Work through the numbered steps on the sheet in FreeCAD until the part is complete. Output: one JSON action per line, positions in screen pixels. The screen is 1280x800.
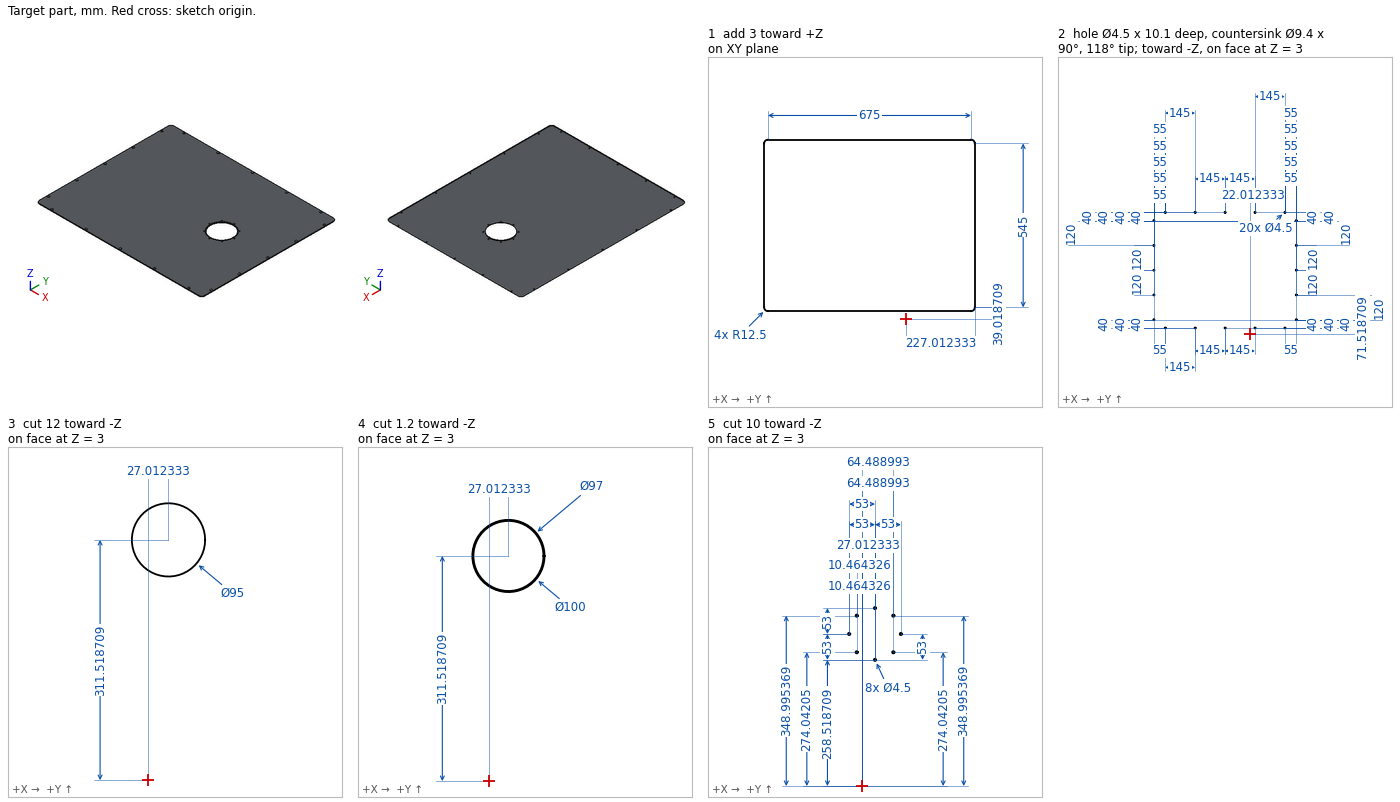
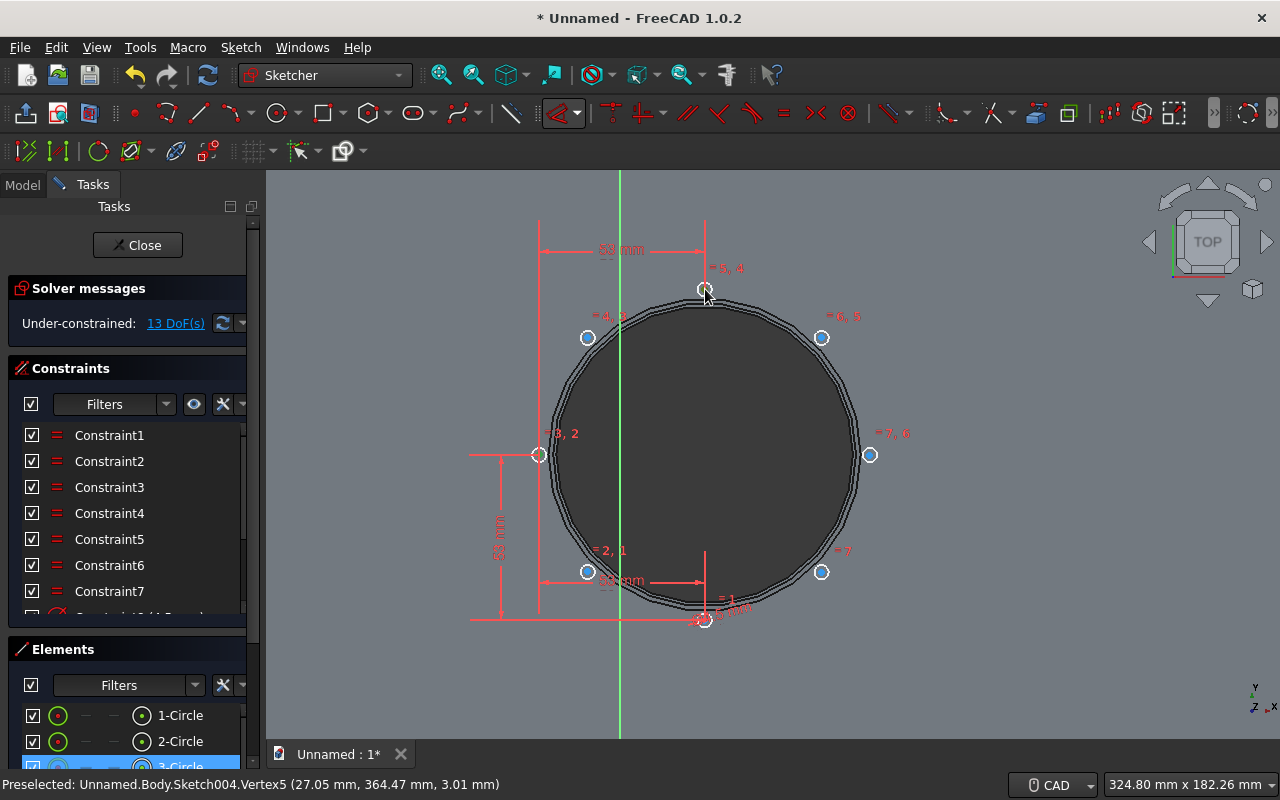
{"action": "left_click", "coordinate": [580, 114]}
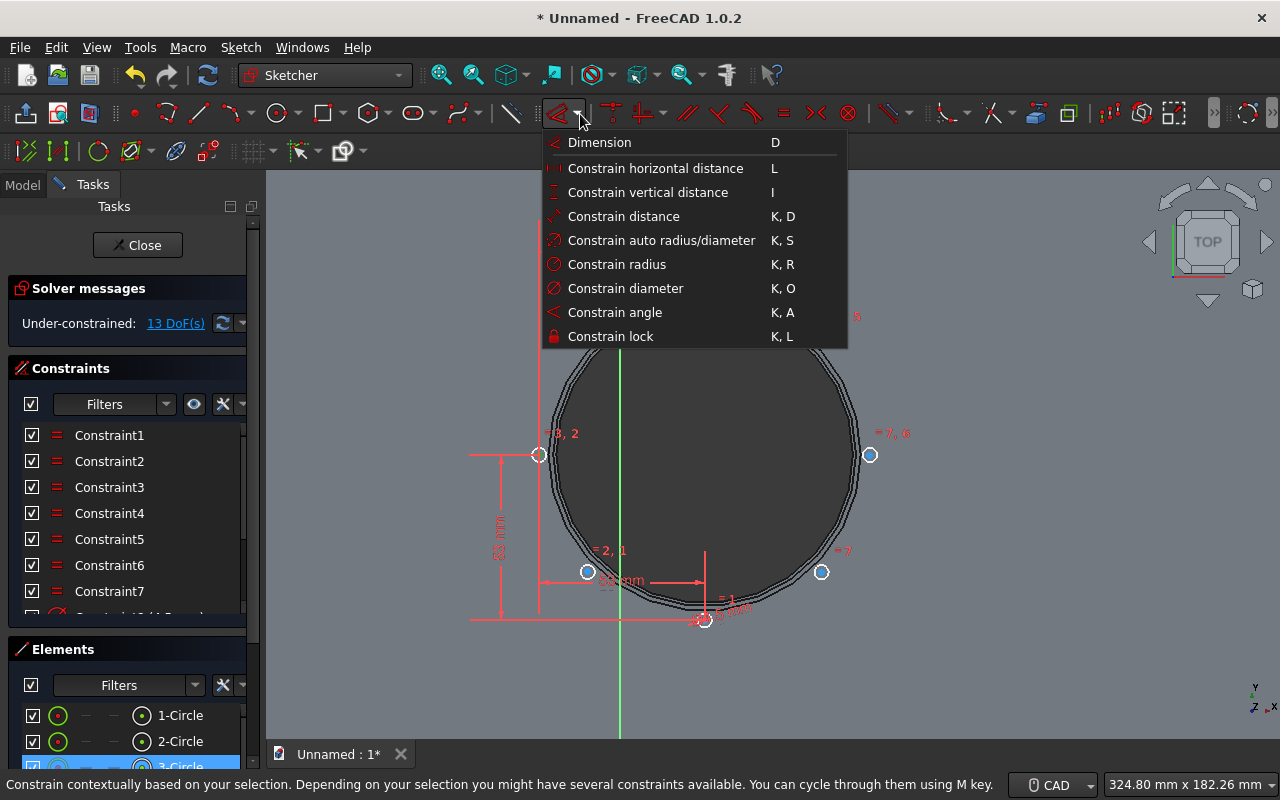
{"action": "left_click", "coordinate": [695, 192]}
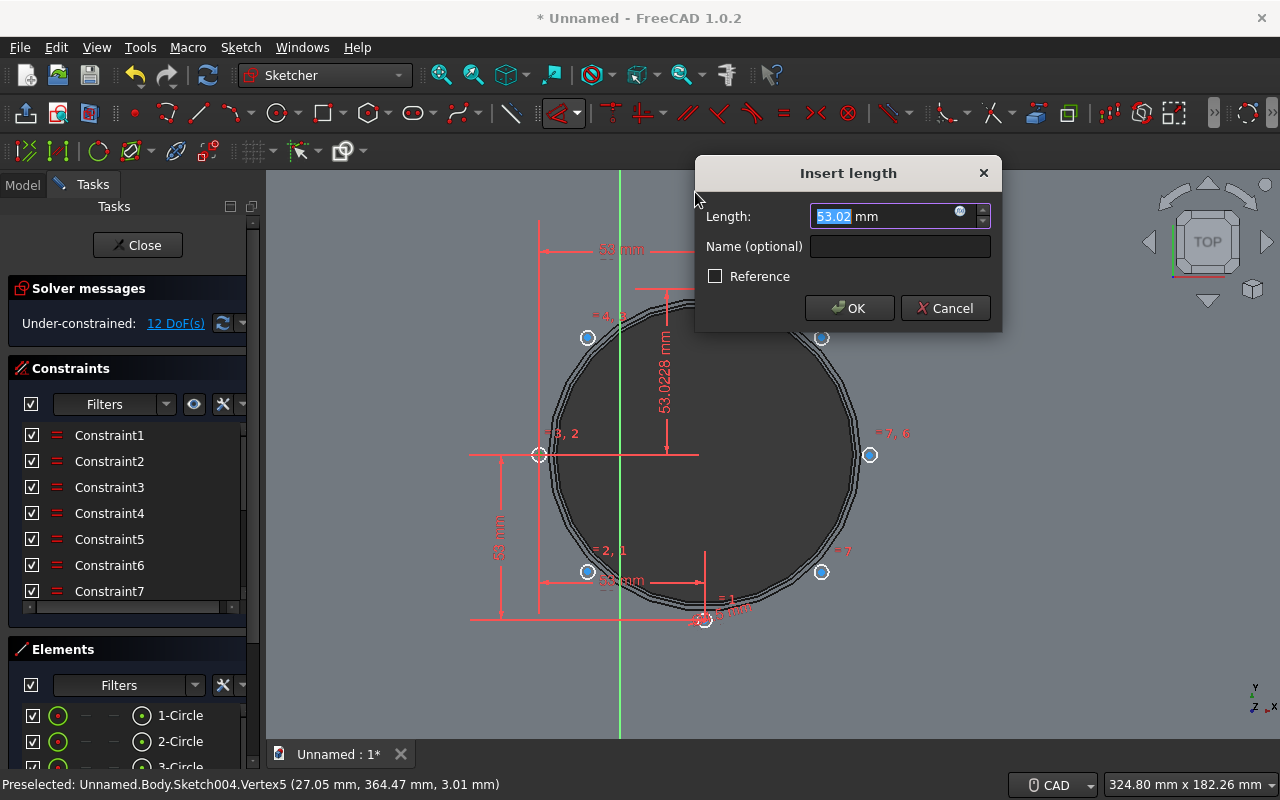
{"action": "type", "text": "53"}
{"action": "key", "text": "Return"}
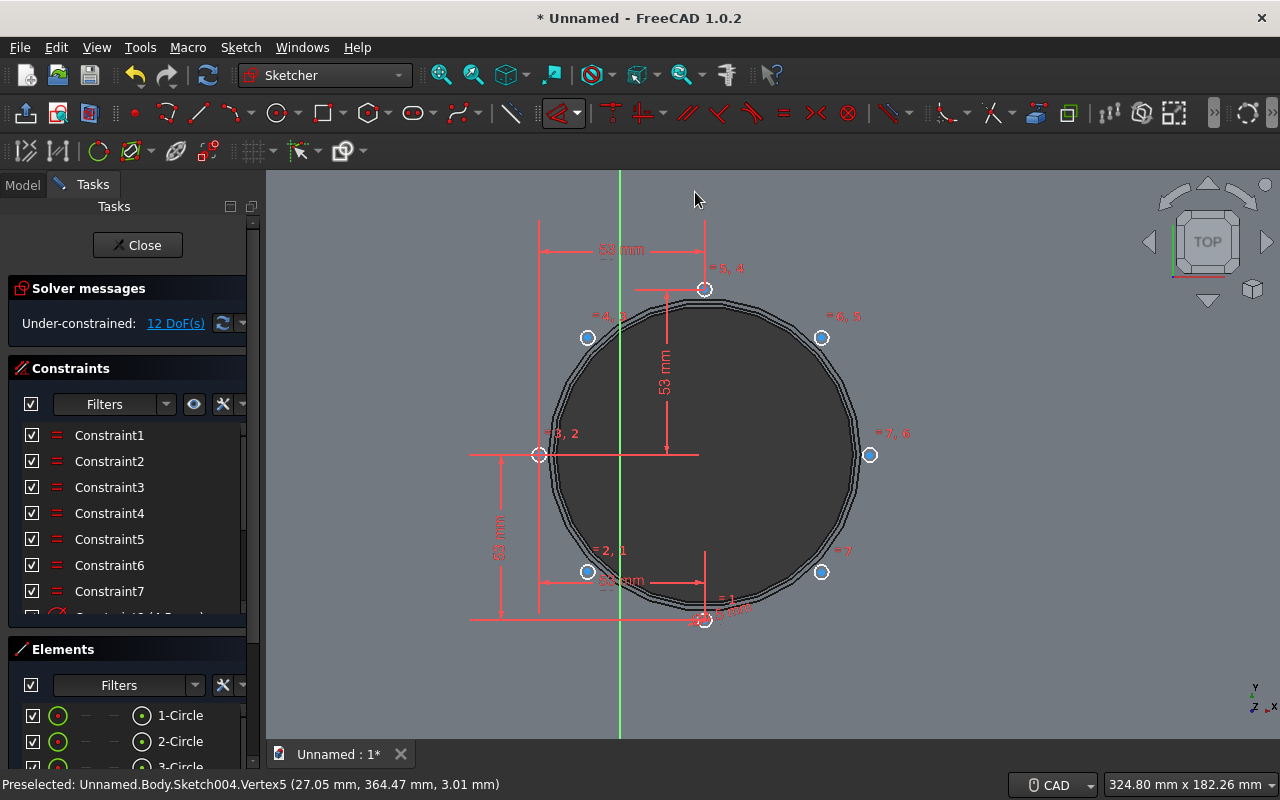
{"action": "left_click", "coordinate": [705, 620]}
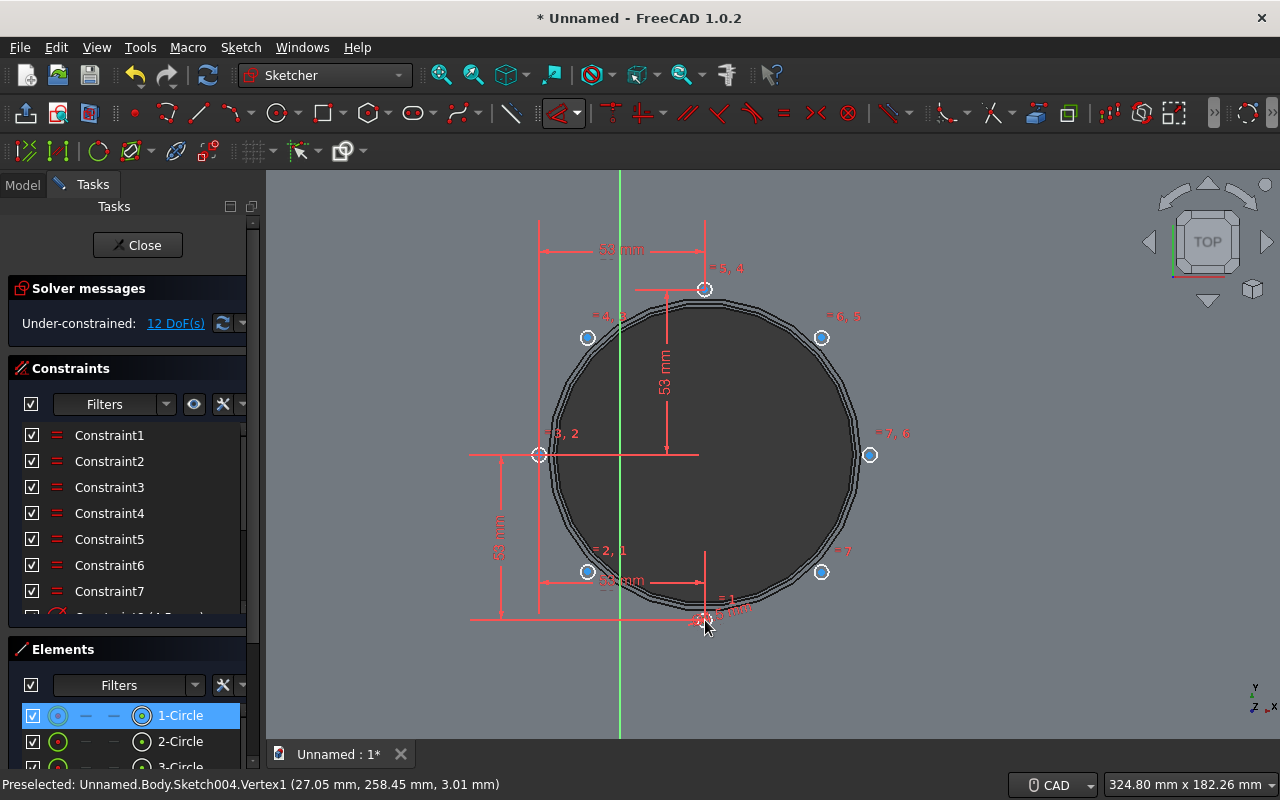
{"action": "left_click", "coordinate": [870, 455]}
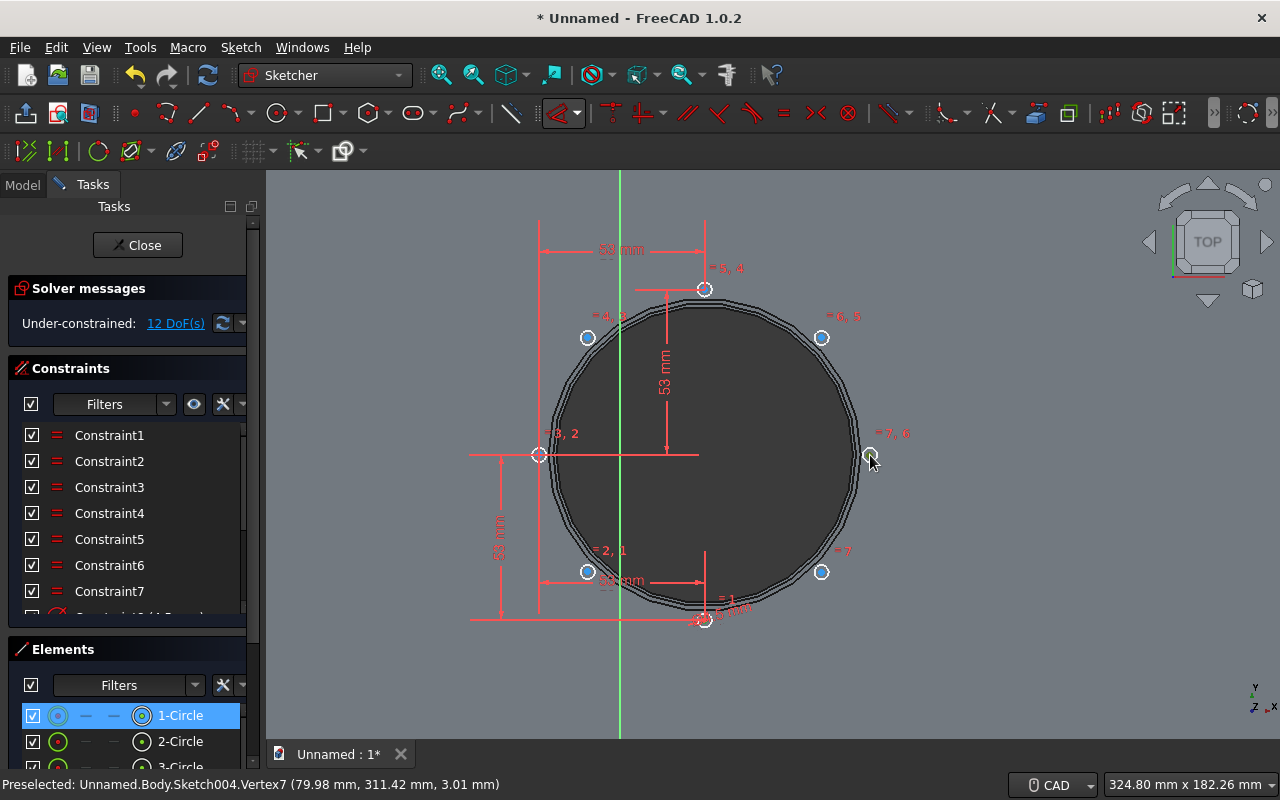
{"action": "left_click", "coordinate": [580, 114]}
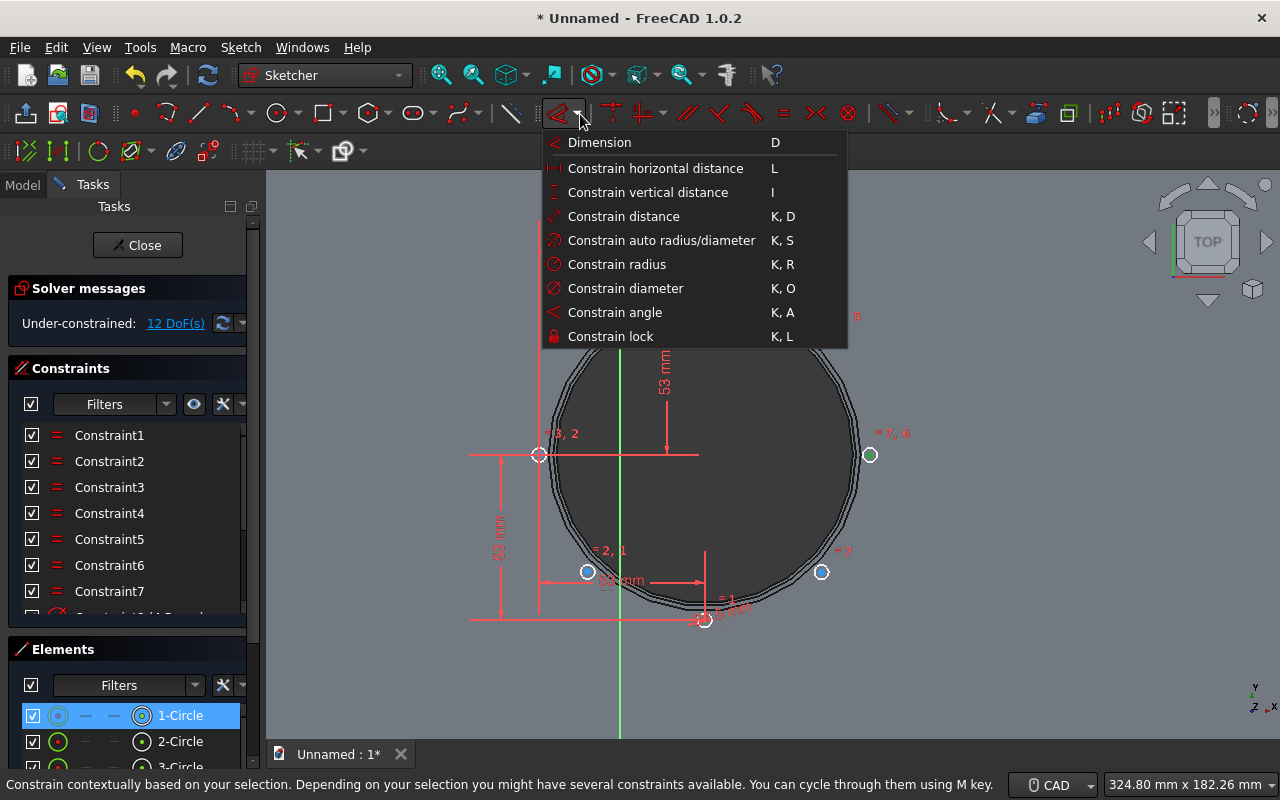
{"action": "left_click", "coordinate": [695, 168]}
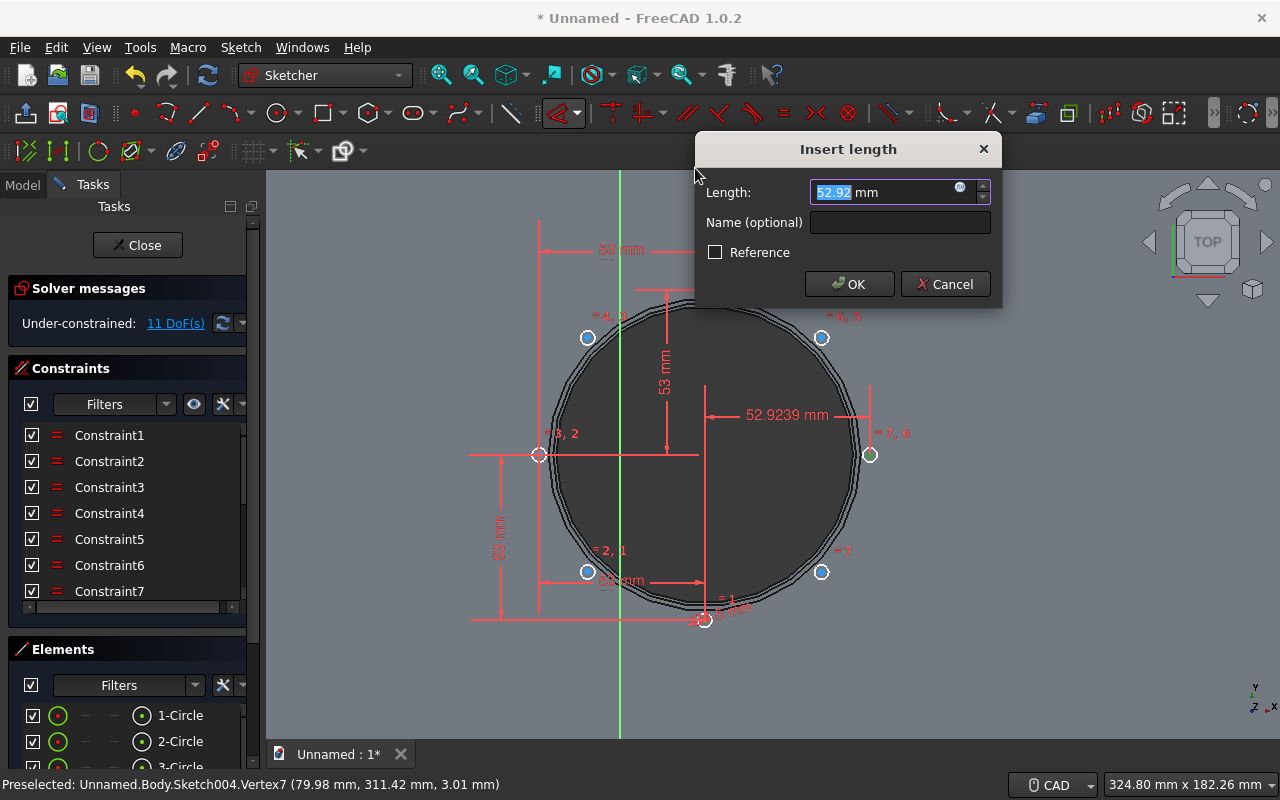
{"action": "type", "text": "53"}
{"action": "key", "text": "Return"}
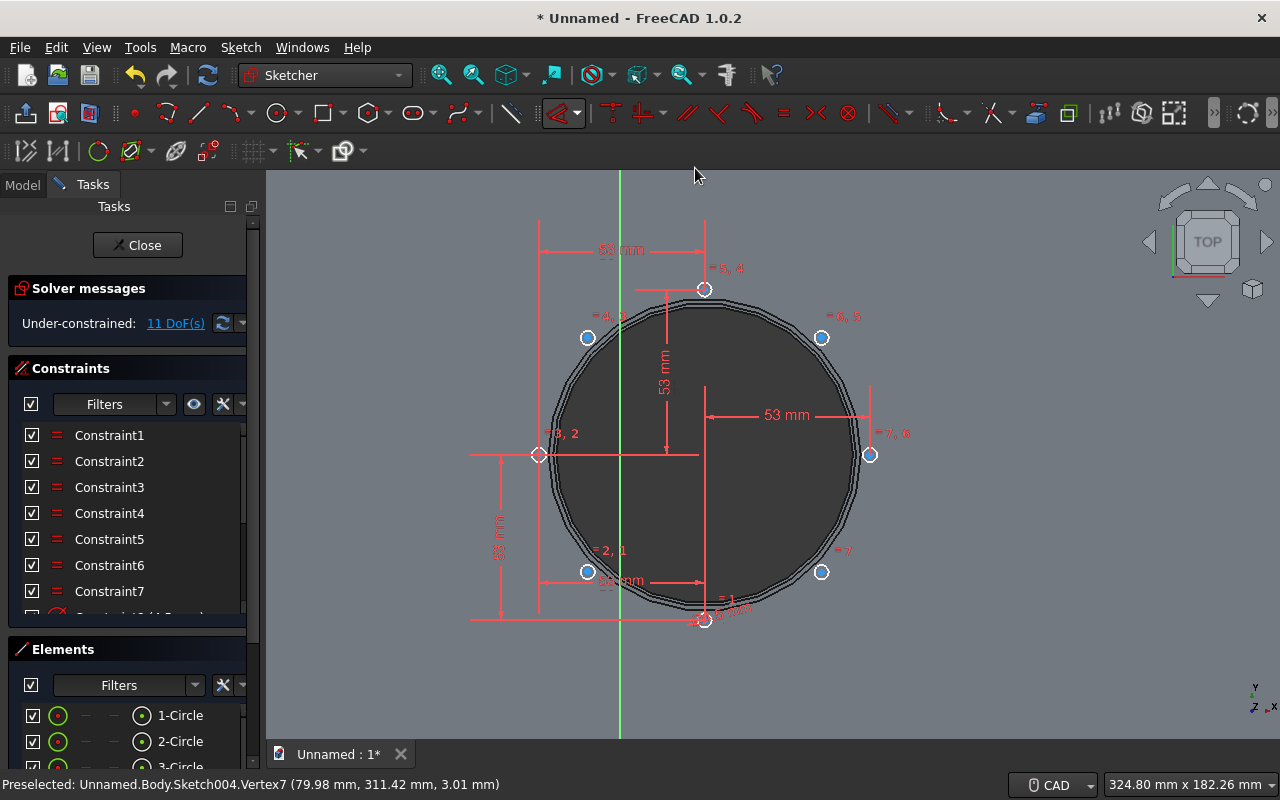
{"action": "left_click", "coordinate": [705, 620]}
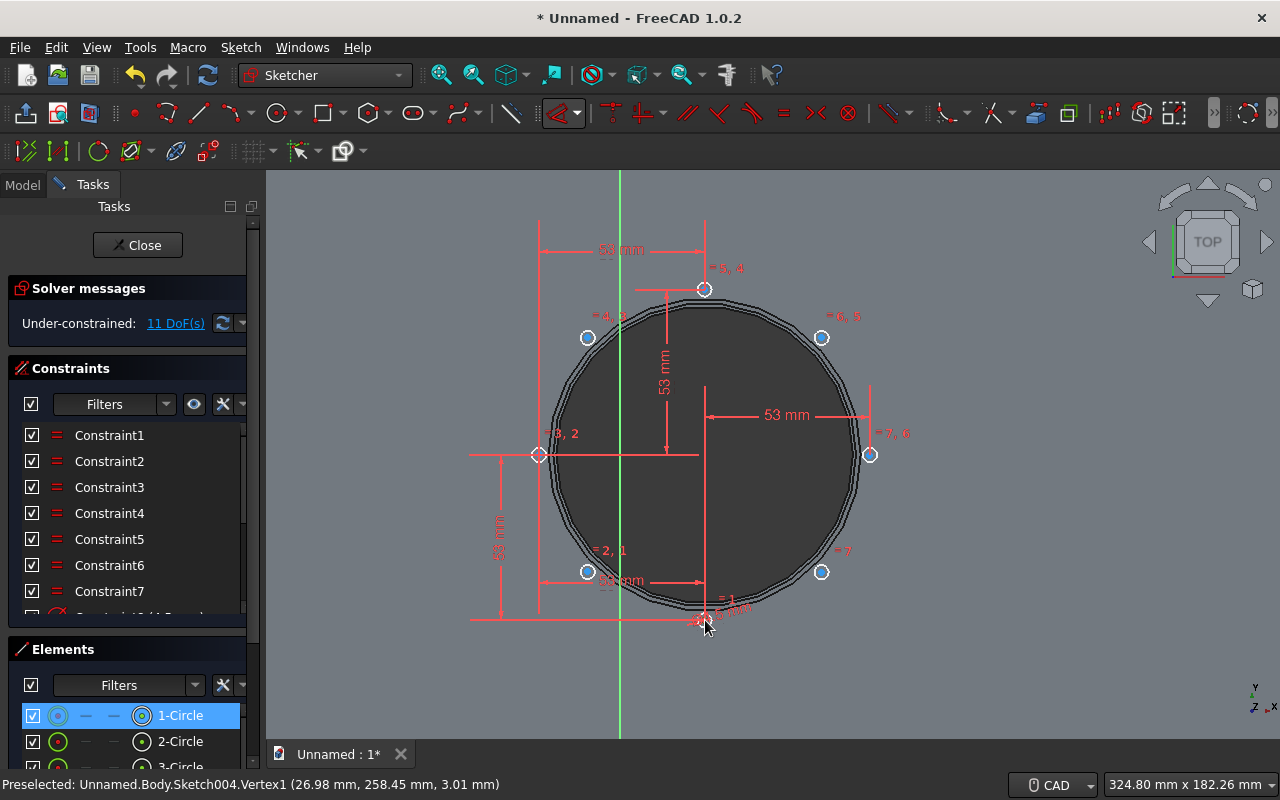
{"action": "left_click", "coordinate": [870, 455]}